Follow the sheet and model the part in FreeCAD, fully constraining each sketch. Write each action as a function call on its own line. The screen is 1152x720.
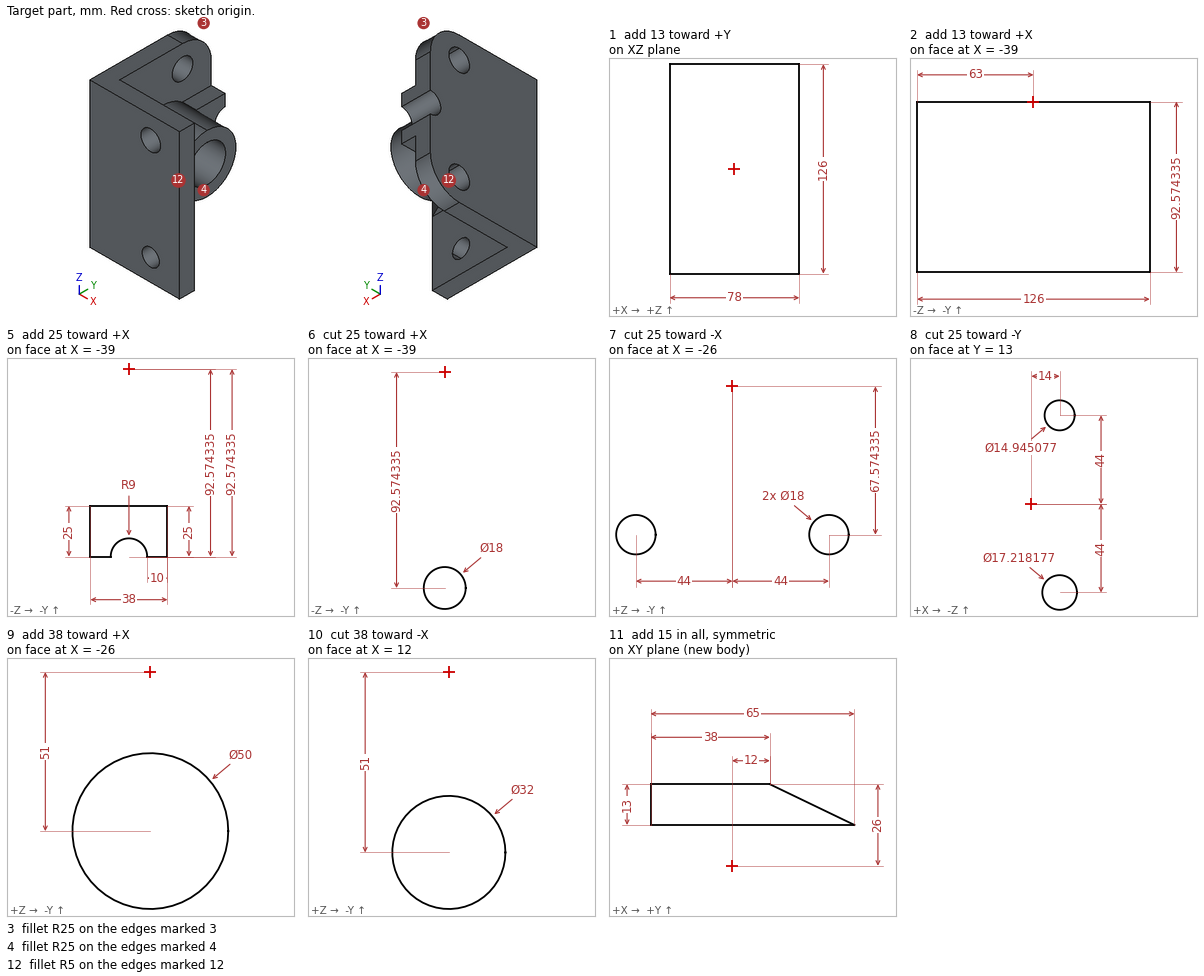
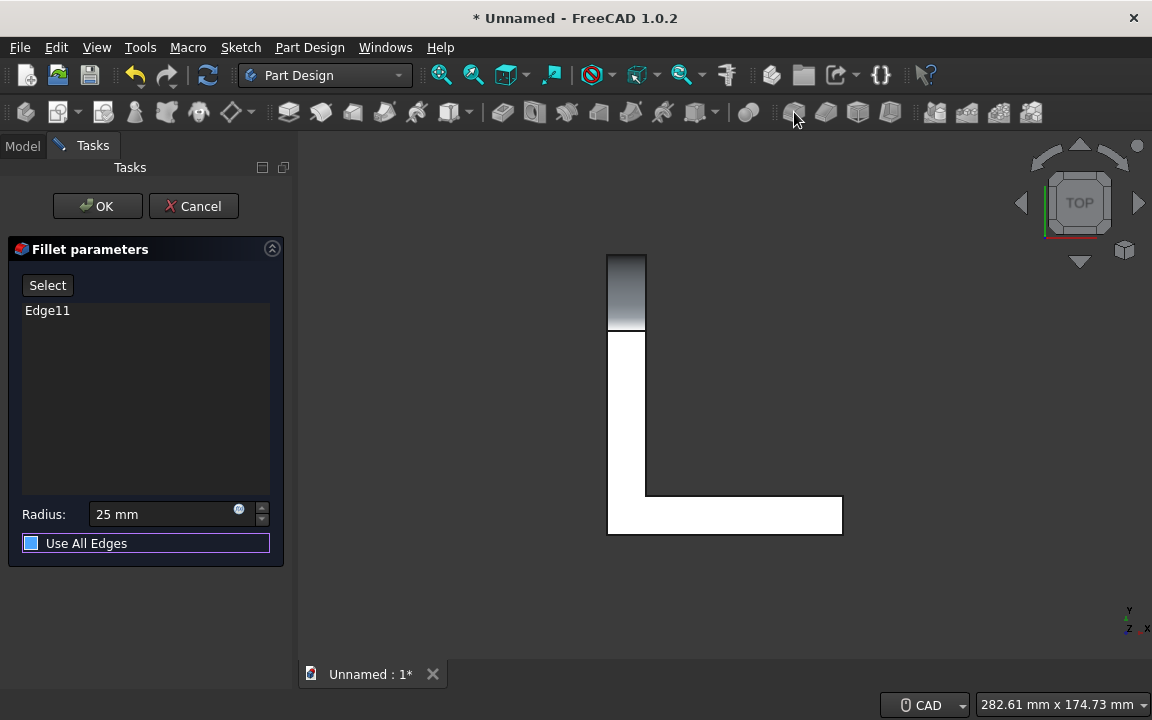
click(98, 206)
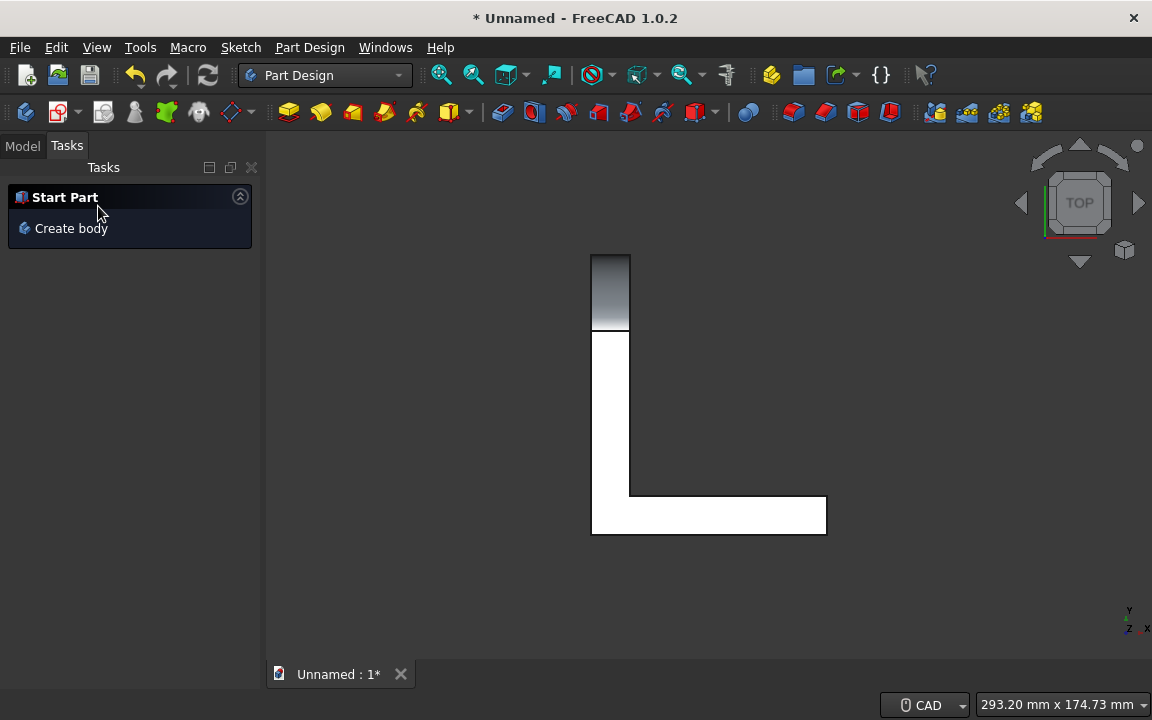
key(0)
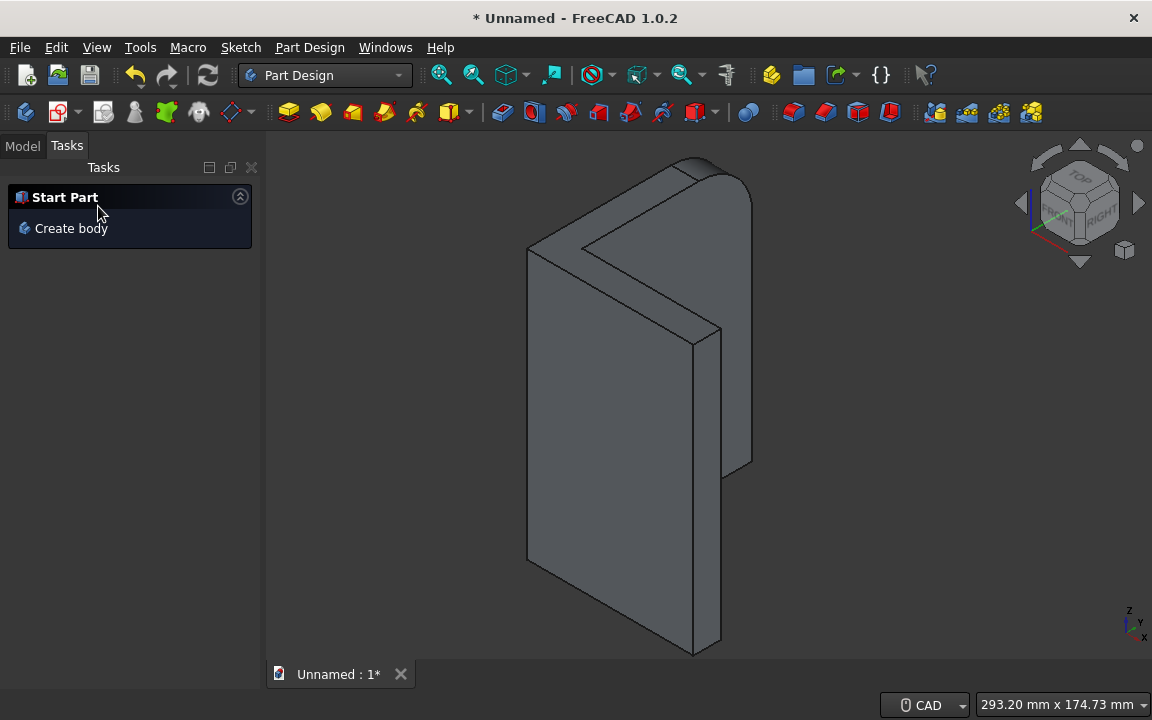
key(2)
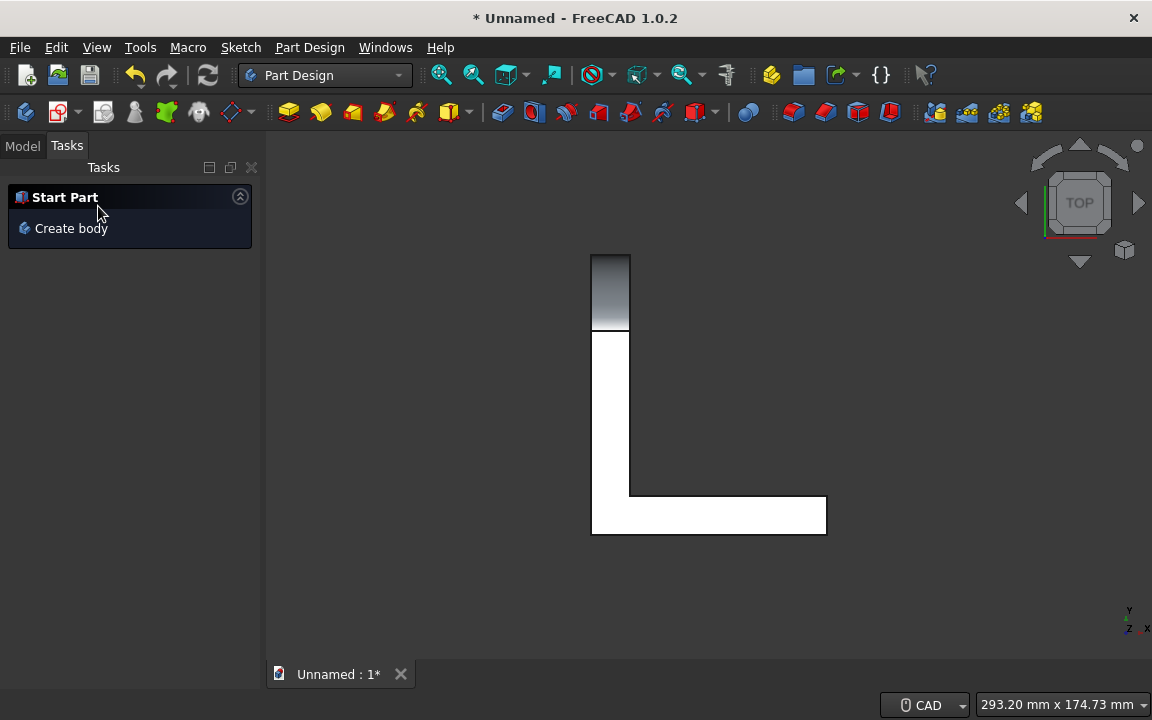
key(1)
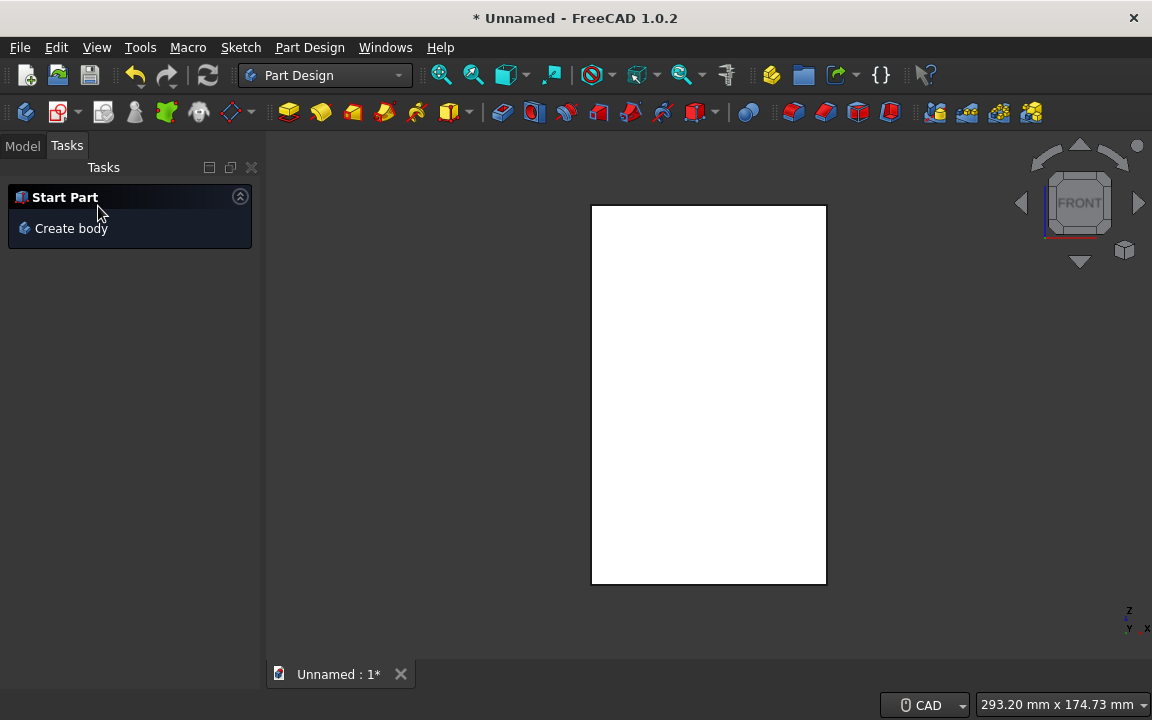
key(3)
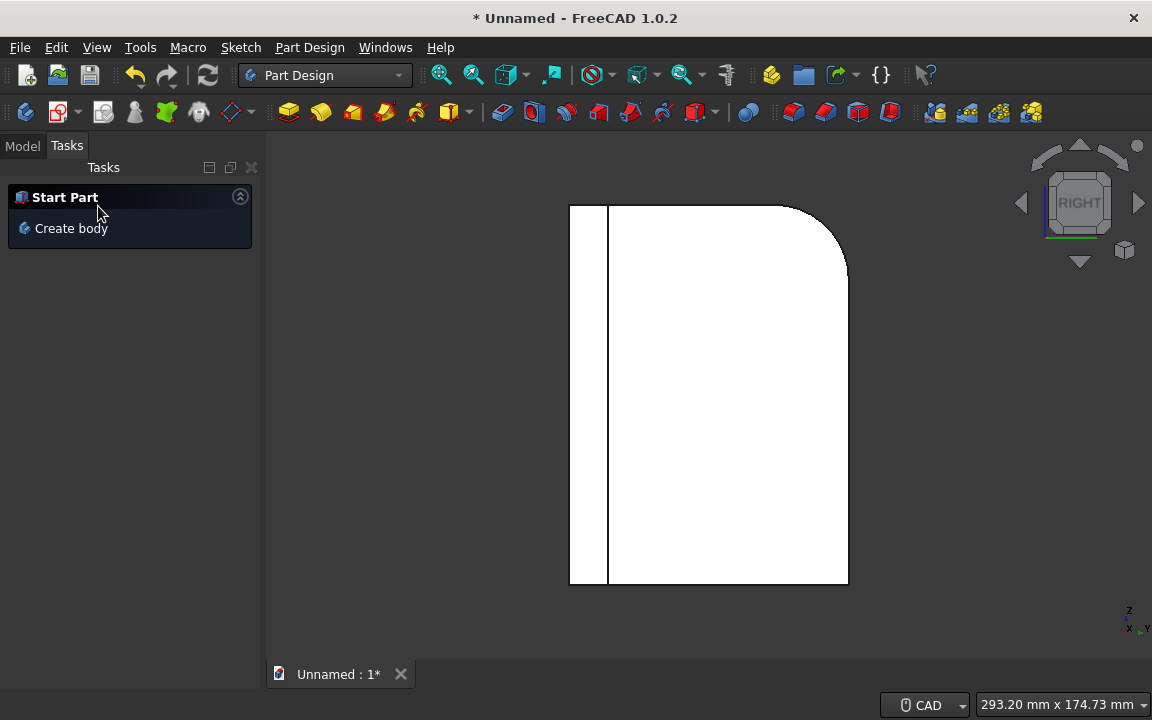
key(5)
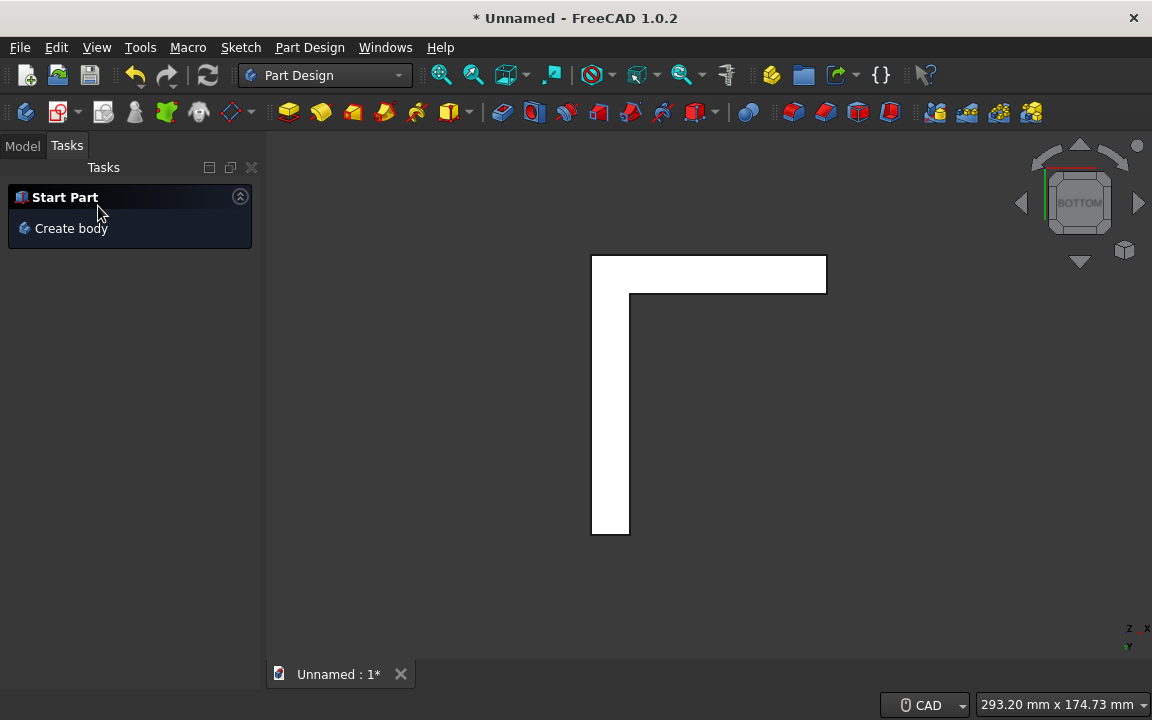
key(4)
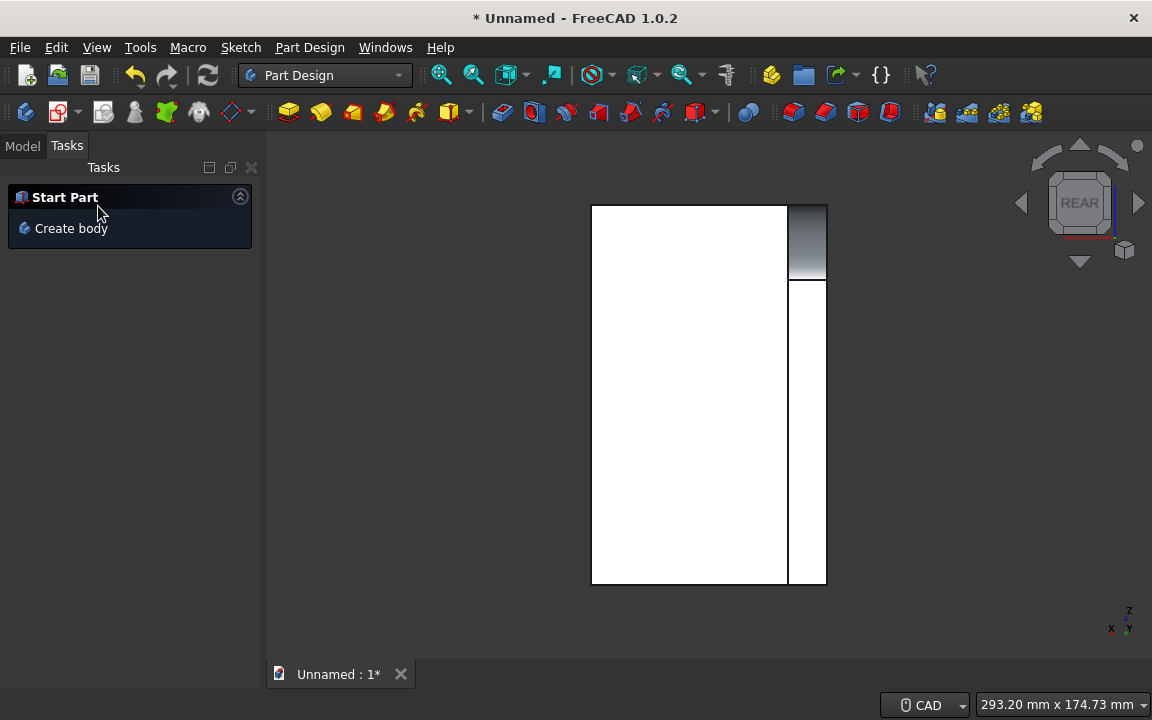
click(807, 584)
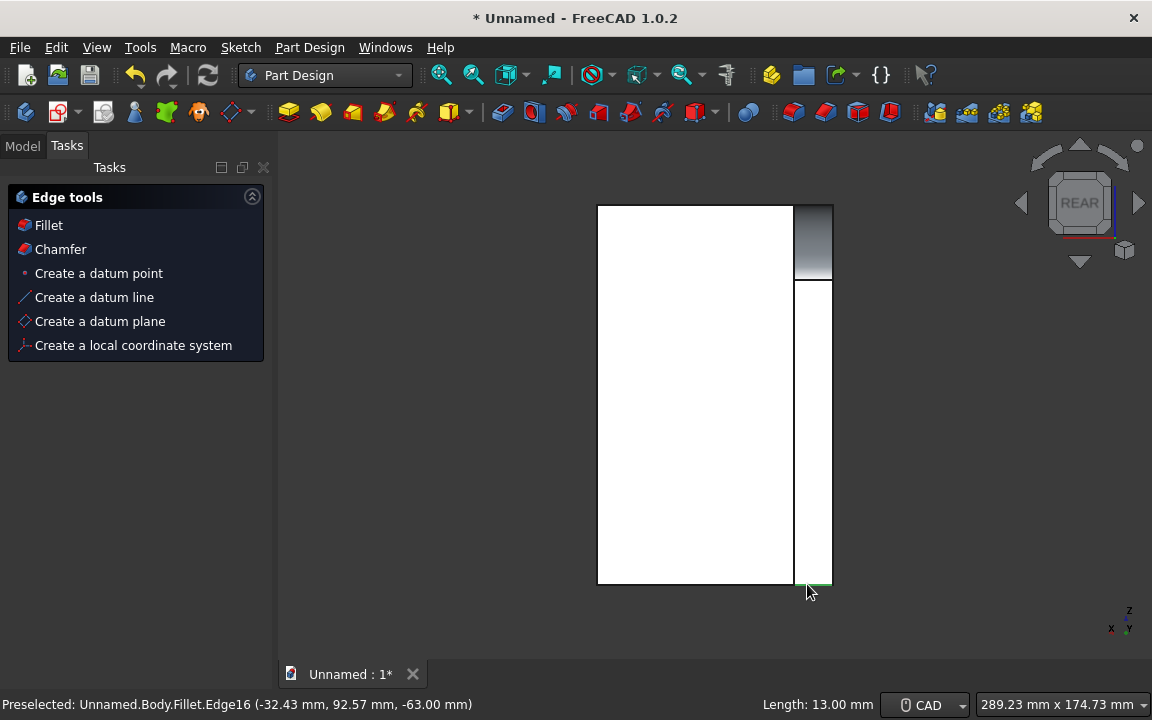
click(794, 112)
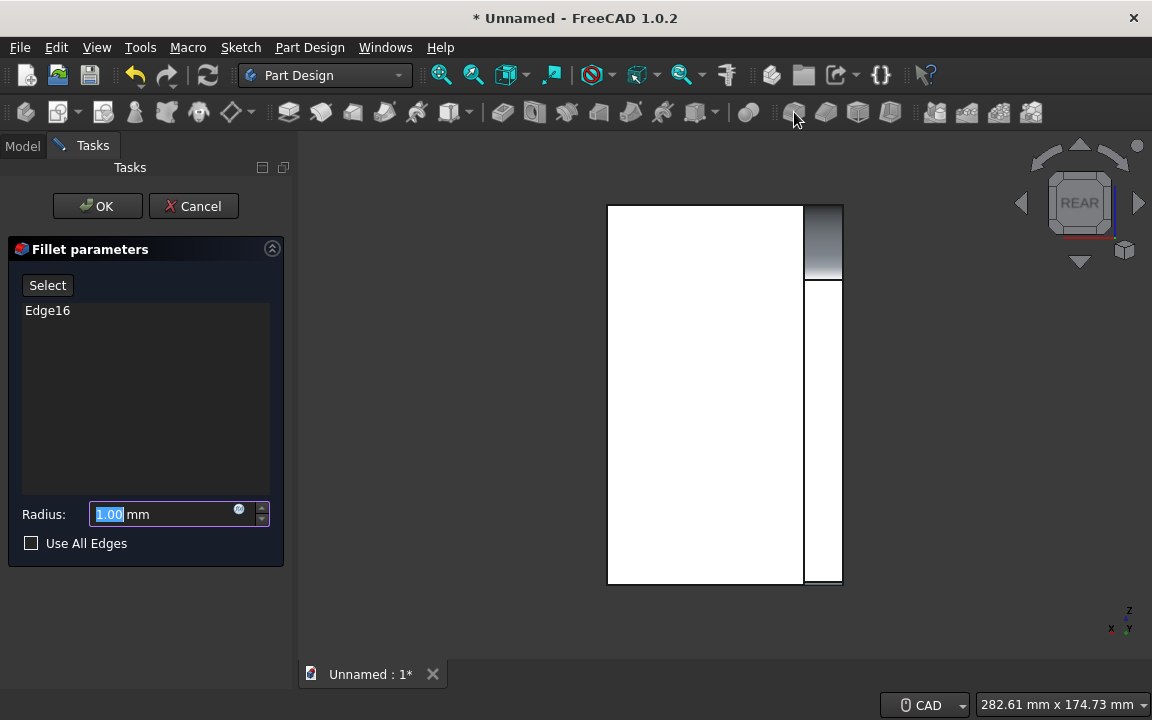
text(25)
key(Tab)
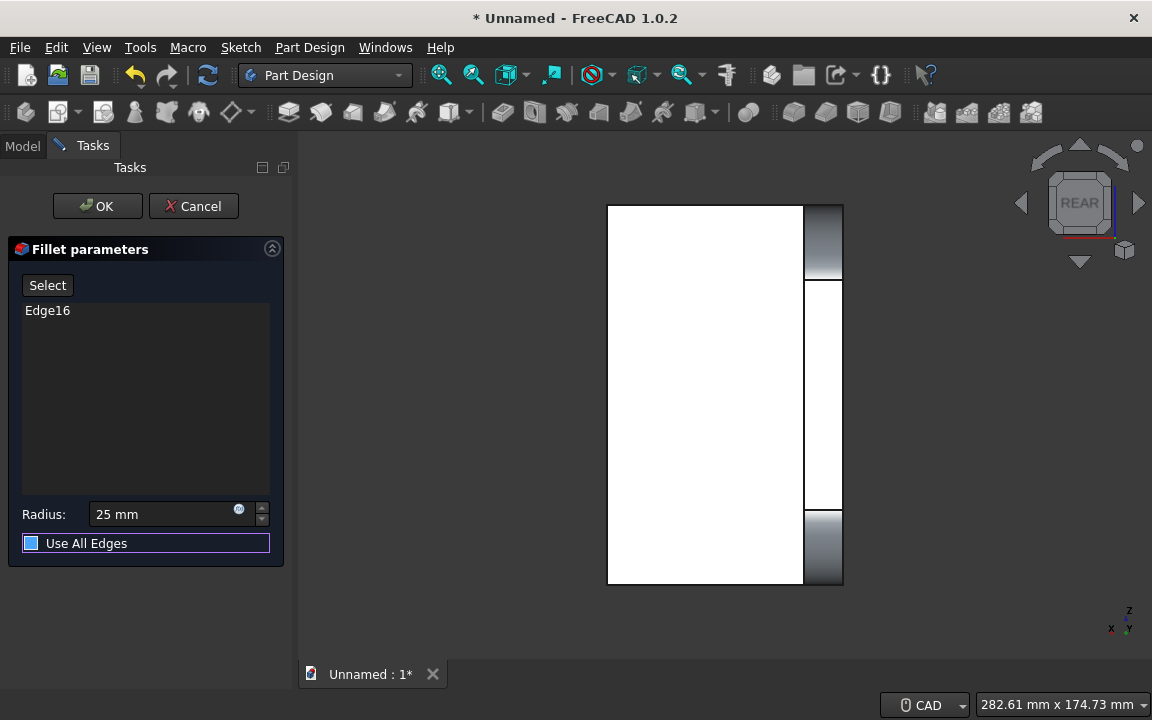
click(98, 206)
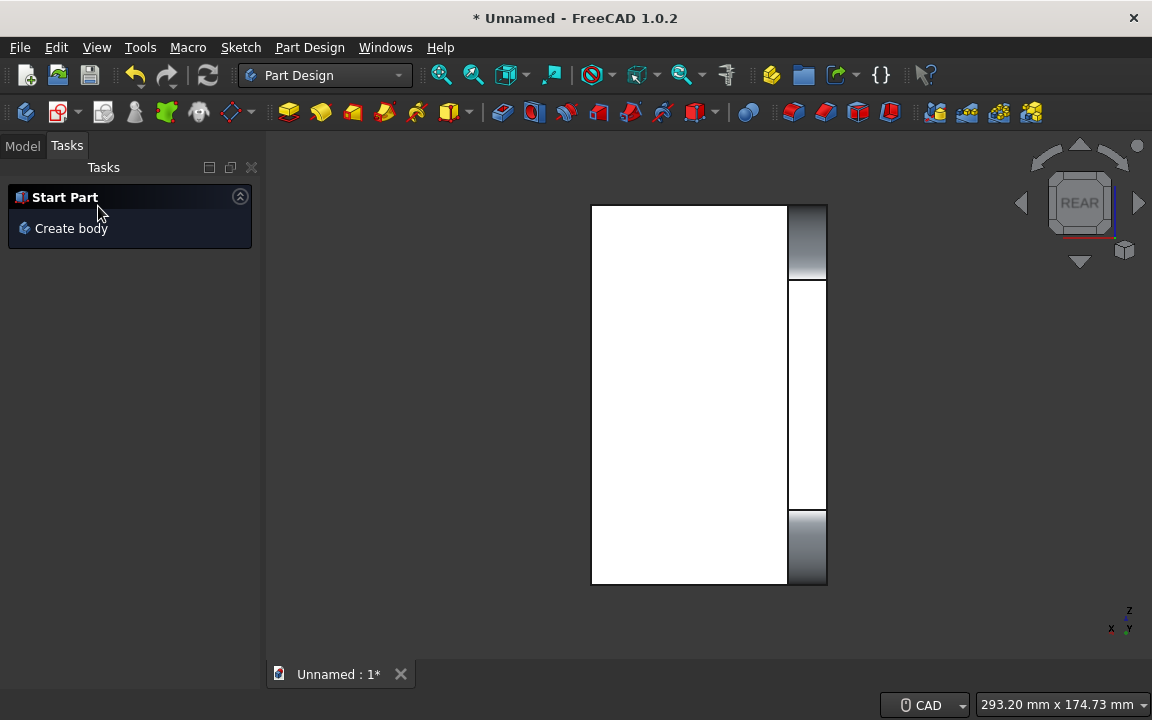
key(6)